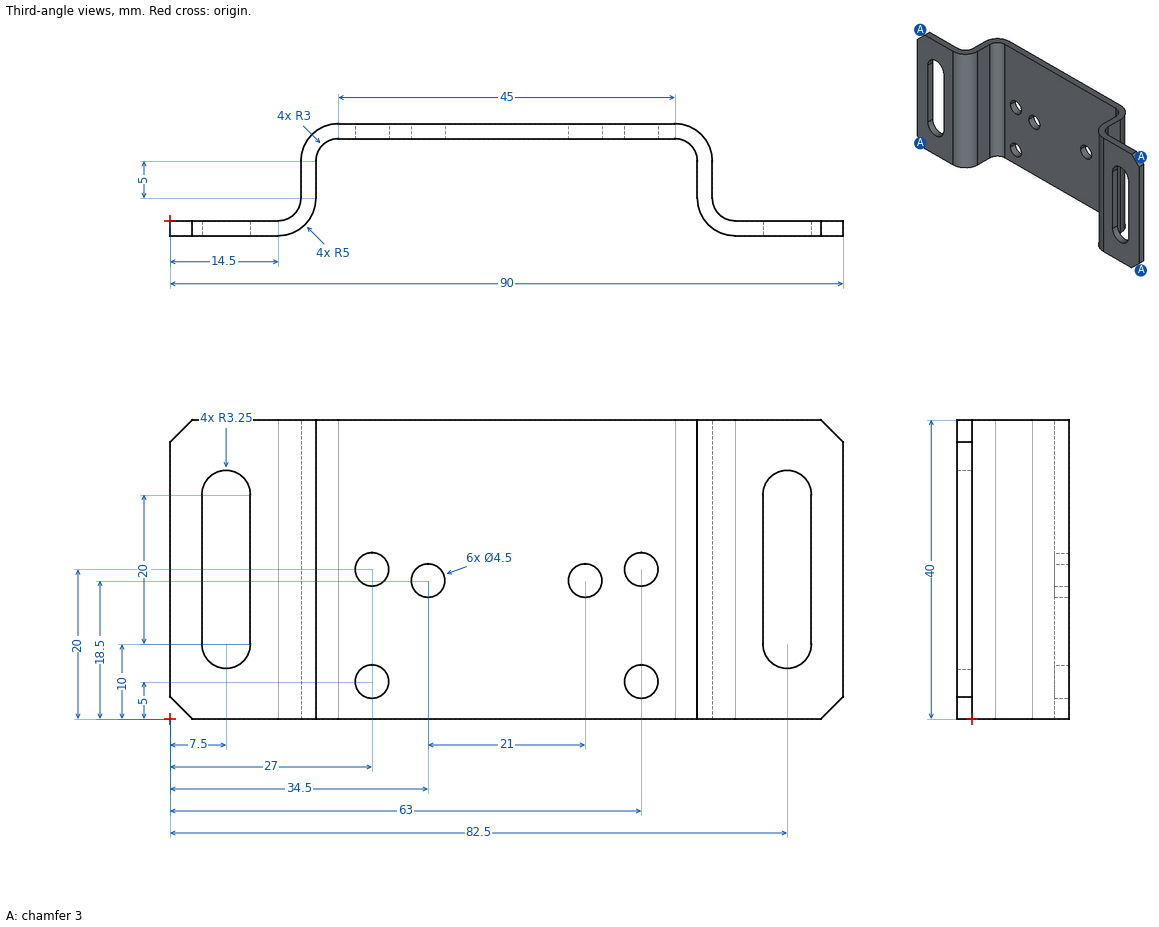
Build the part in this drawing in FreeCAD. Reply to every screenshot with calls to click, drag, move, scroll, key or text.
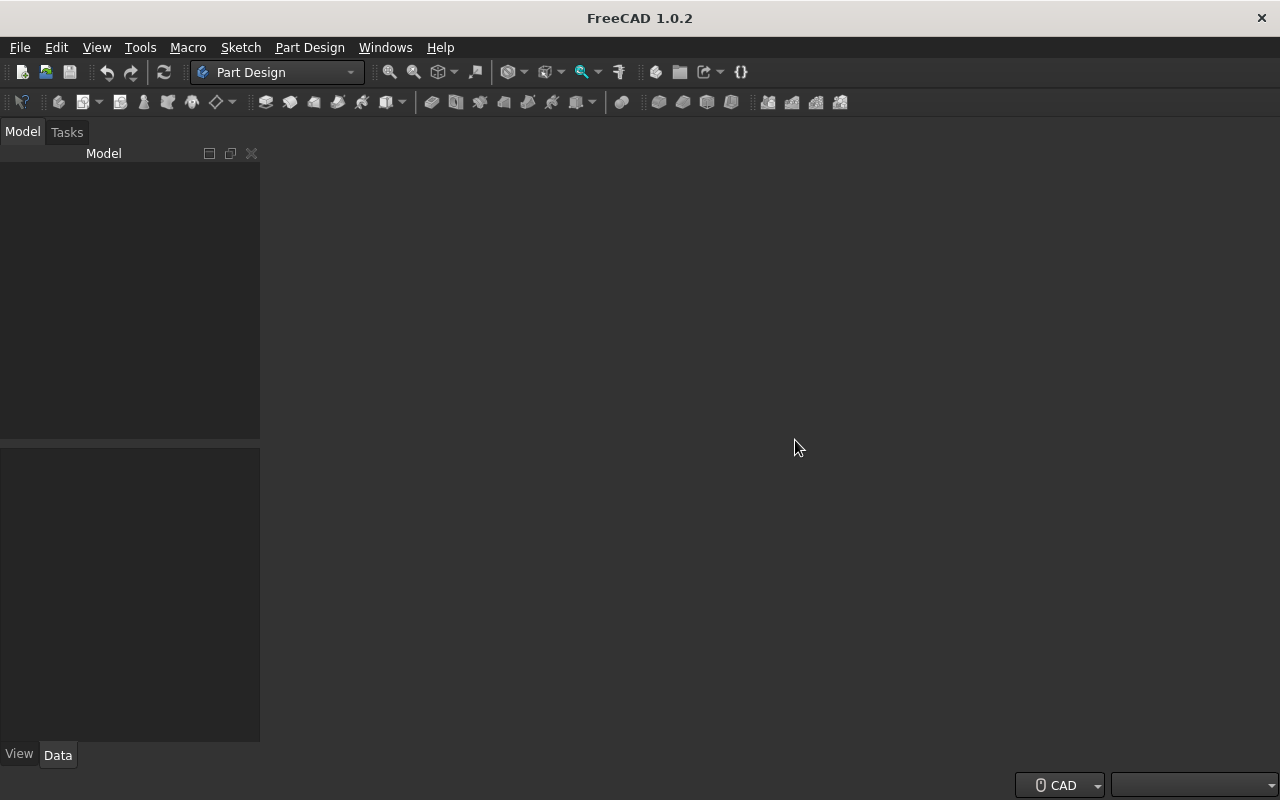
key(ctrl+n)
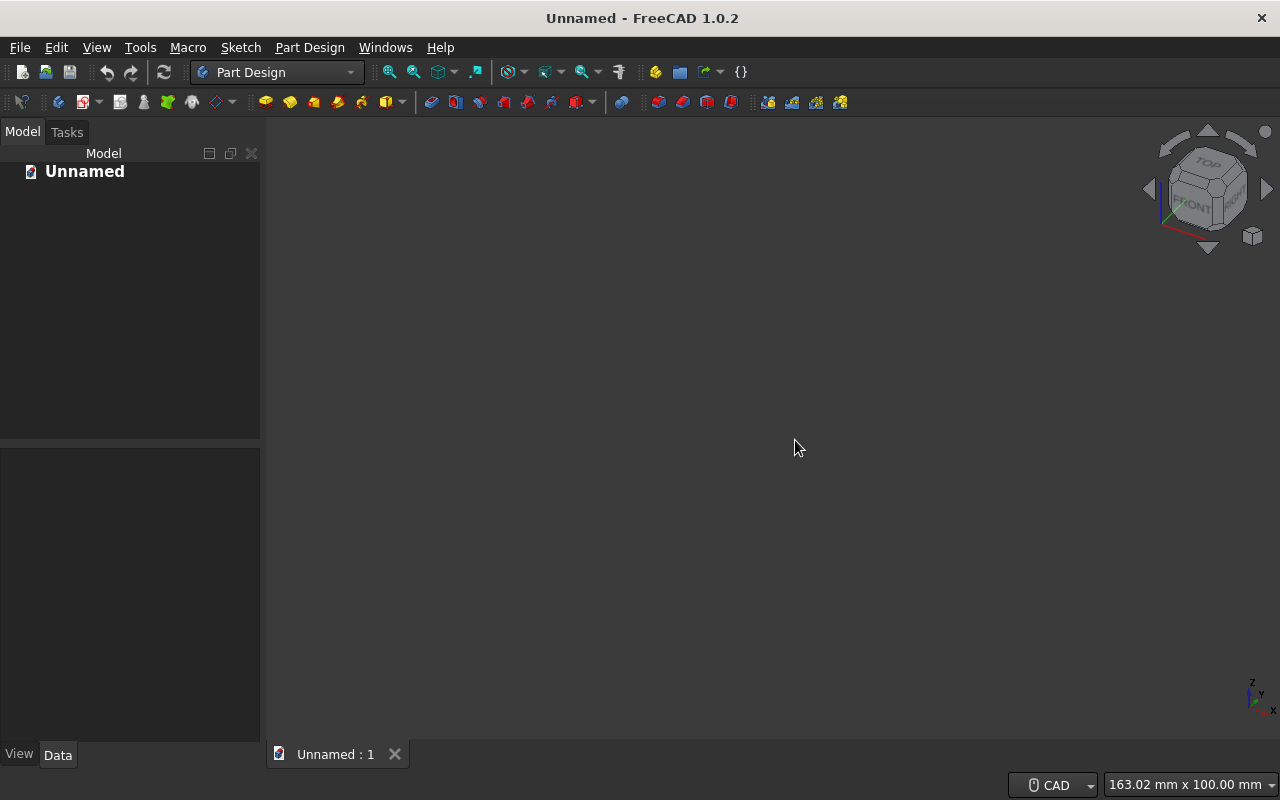
click(84, 102)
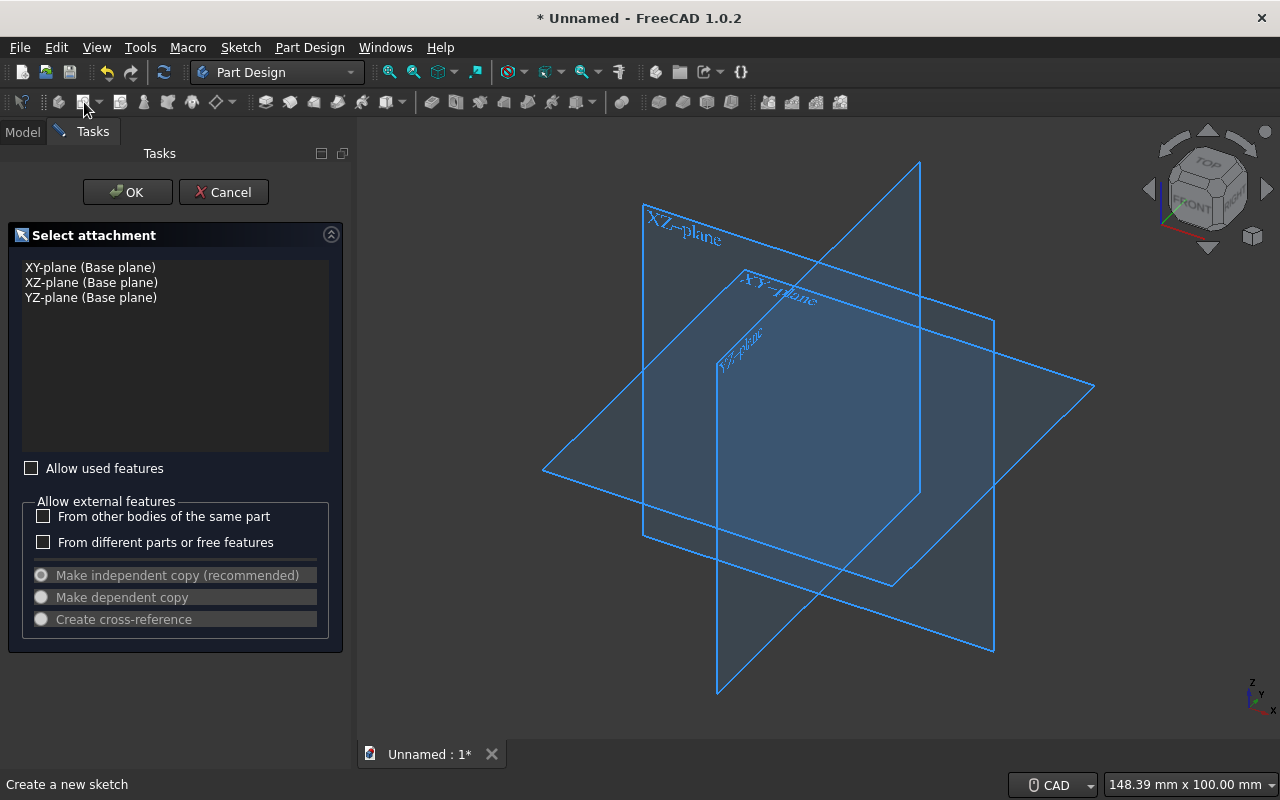
click(82, 268)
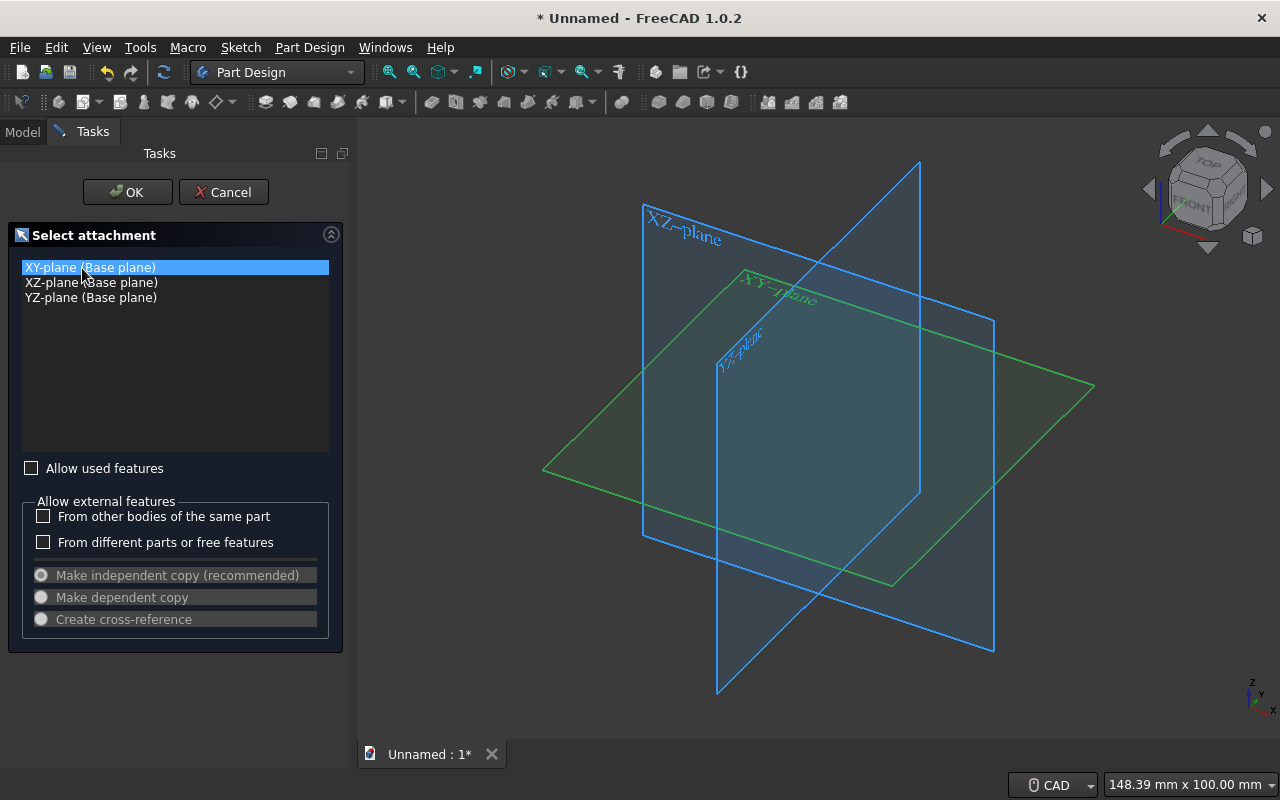
click(128, 192)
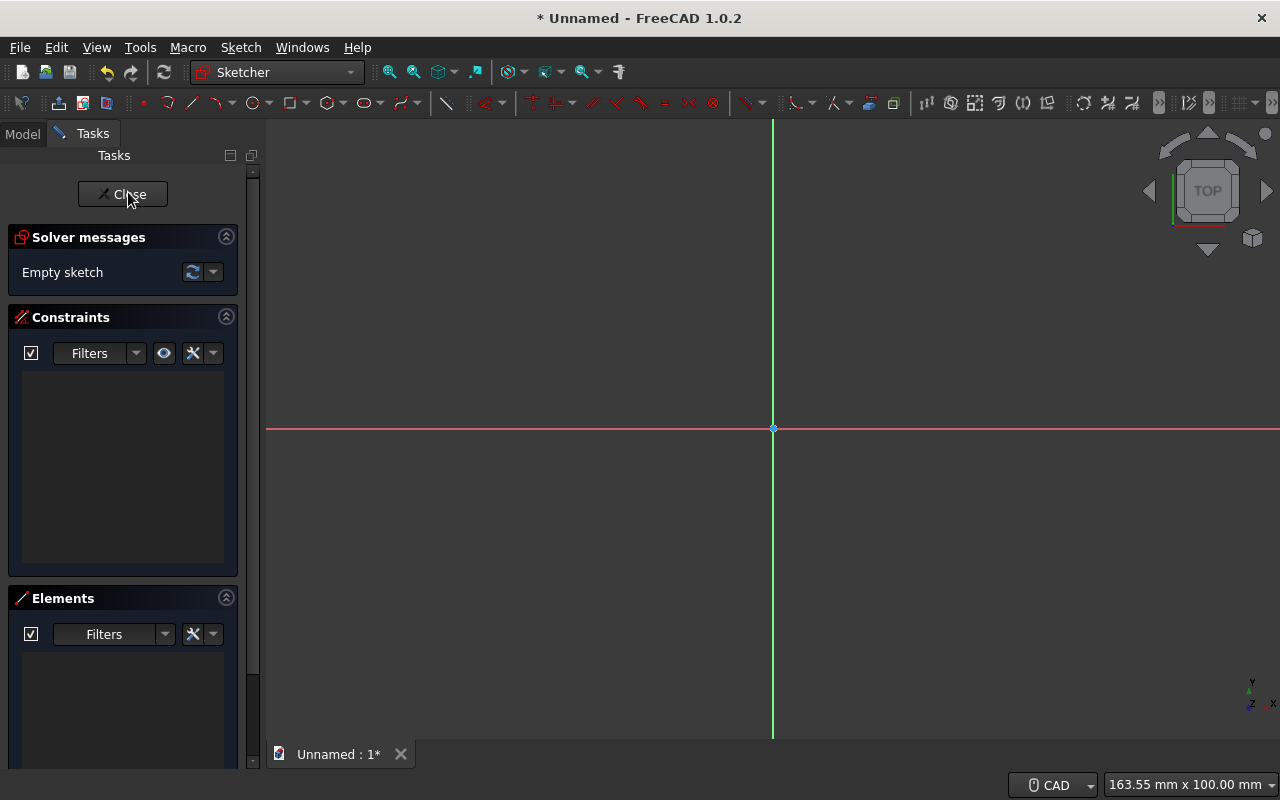
scroll(294, 498, down, 2)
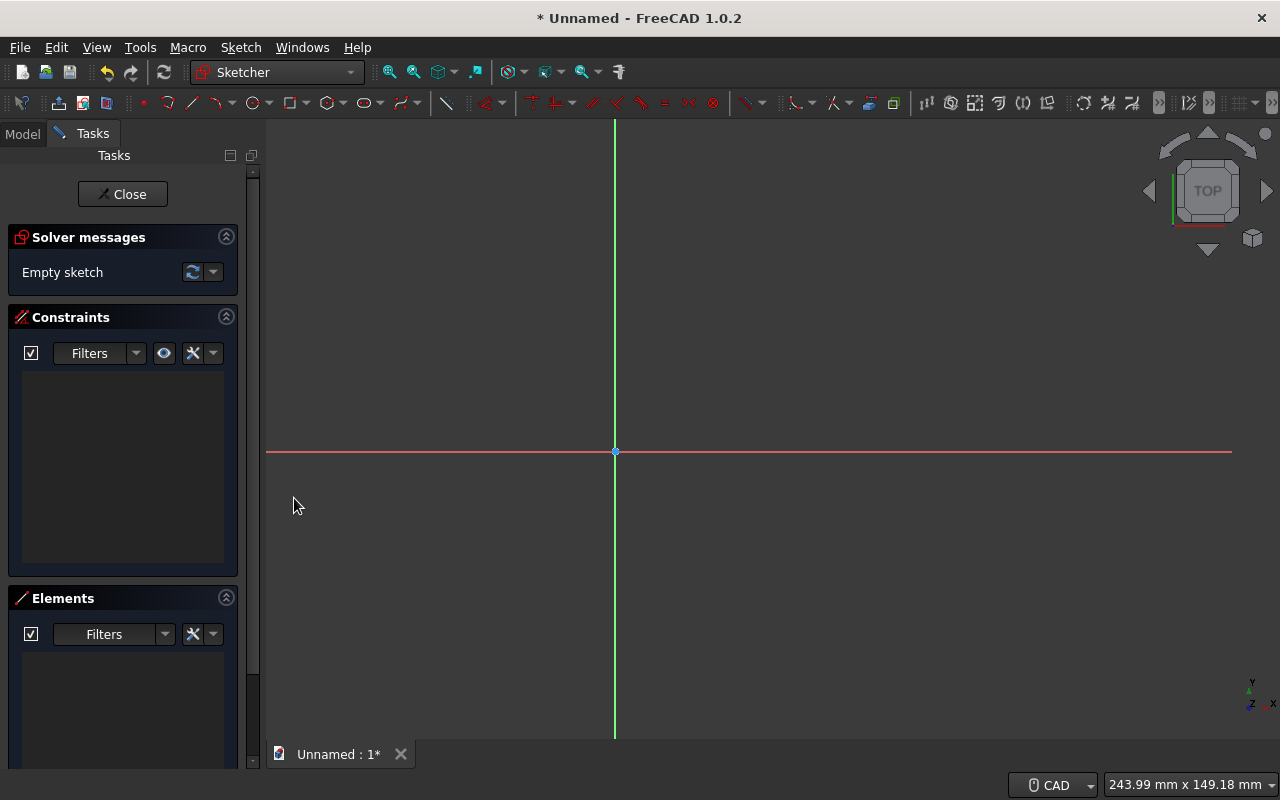
scroll(1001, 429, up, 2)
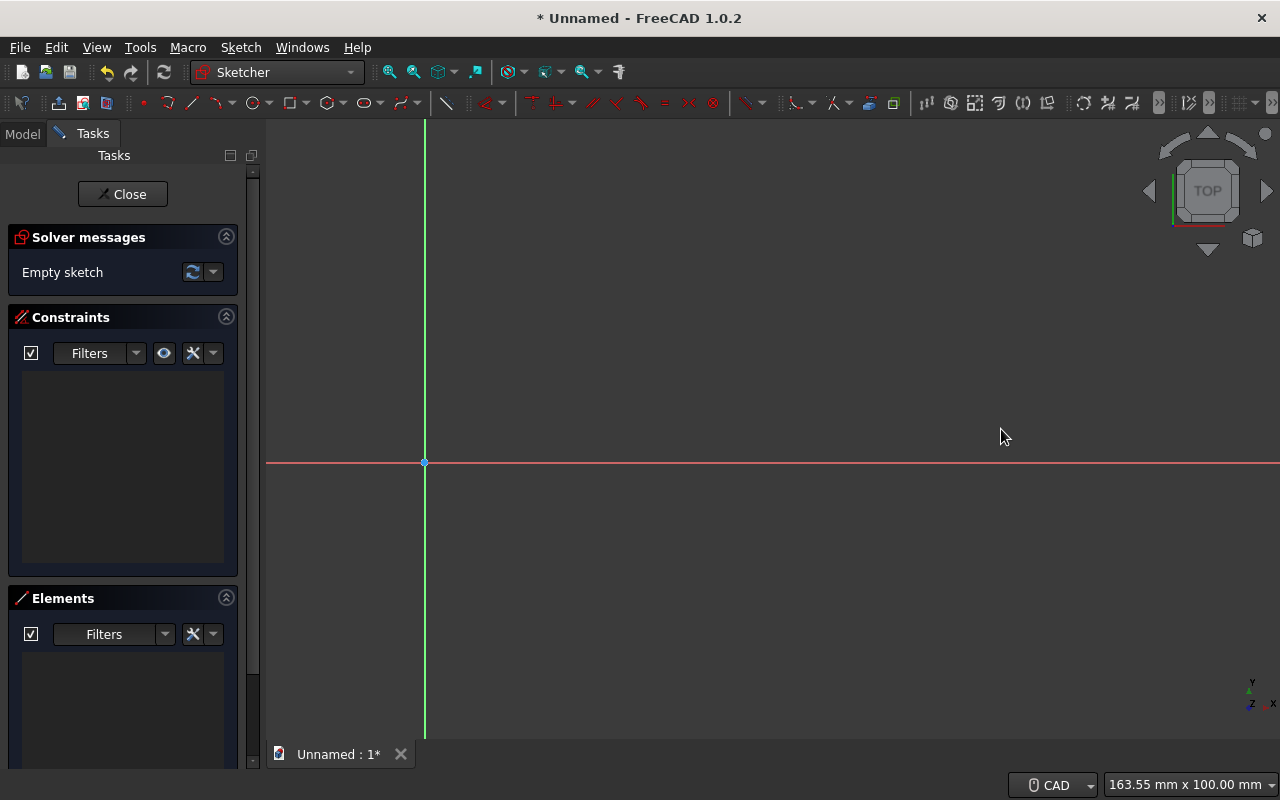
key(g)
key(m)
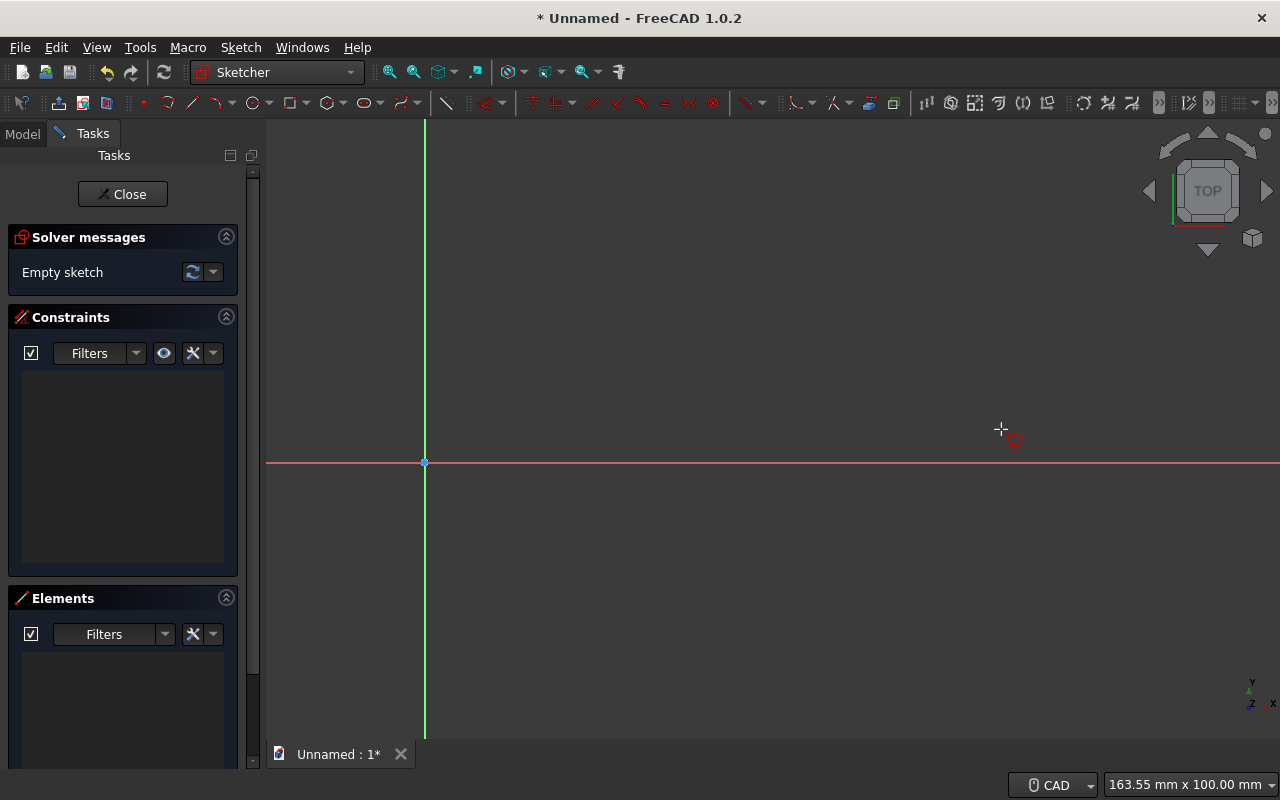
click(515, 463)
click(425, 463)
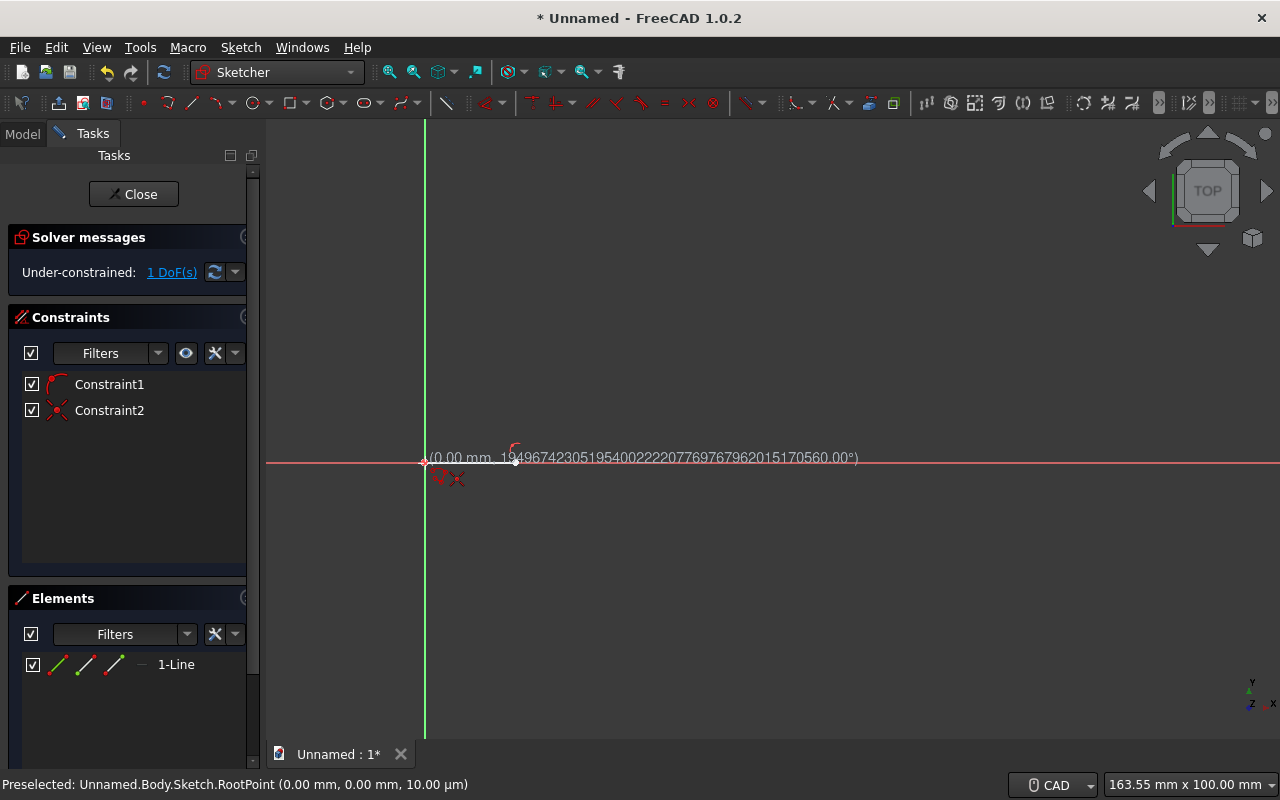
scroll(425, 475, up, 2)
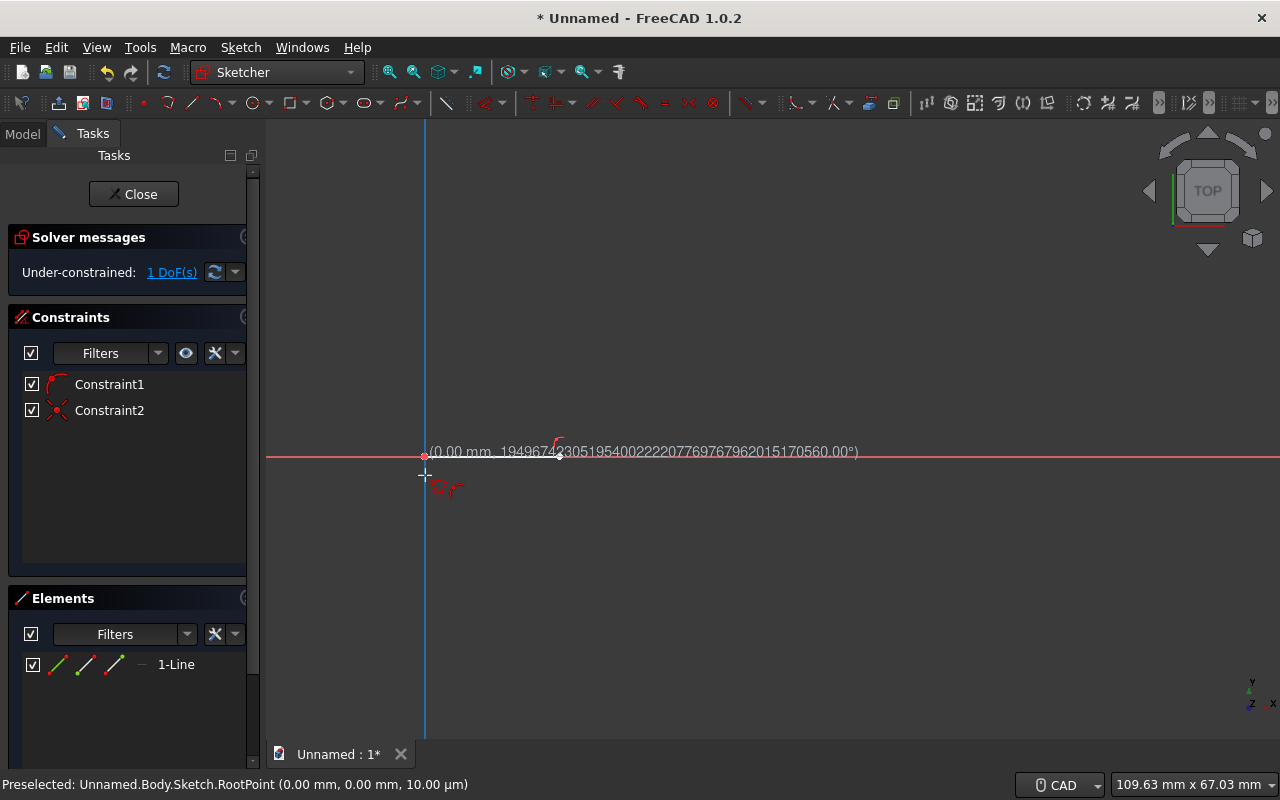
click(434, 475)
click(559, 475)
right_click(559, 475)